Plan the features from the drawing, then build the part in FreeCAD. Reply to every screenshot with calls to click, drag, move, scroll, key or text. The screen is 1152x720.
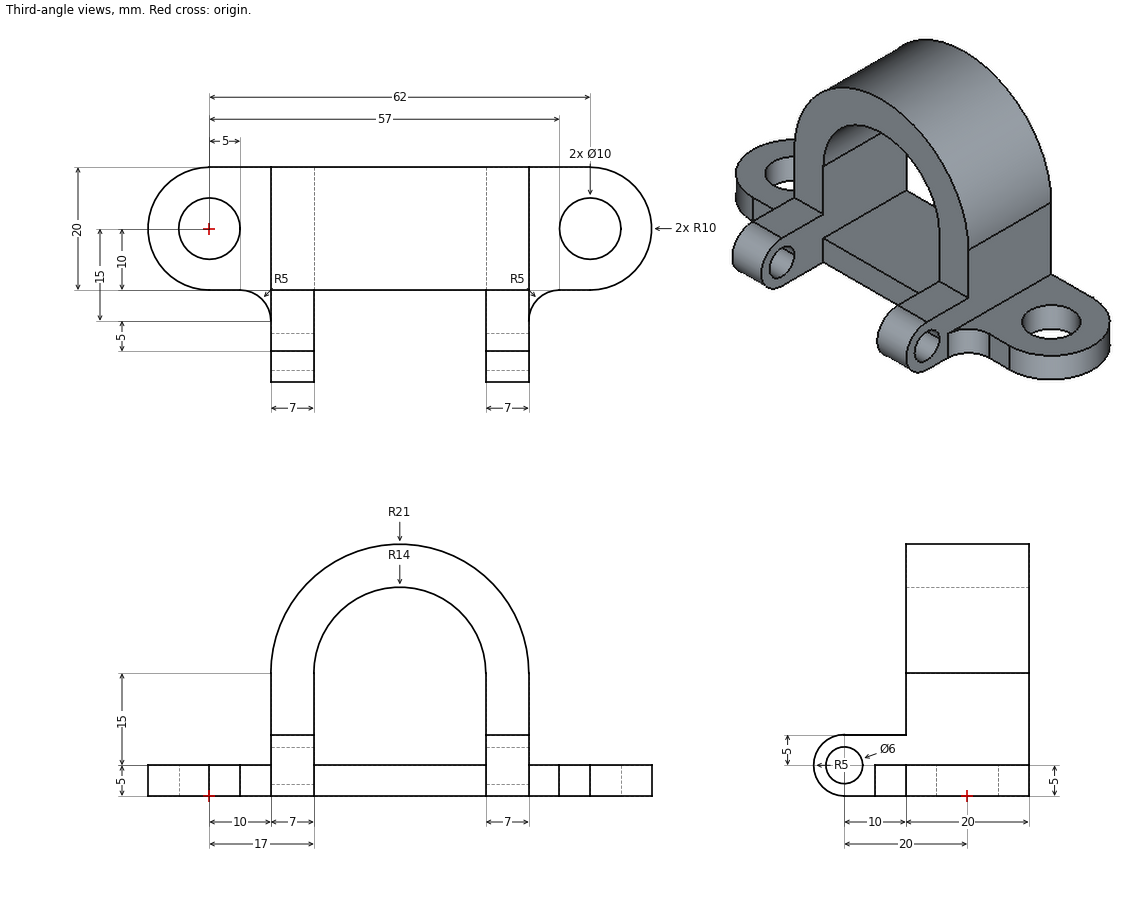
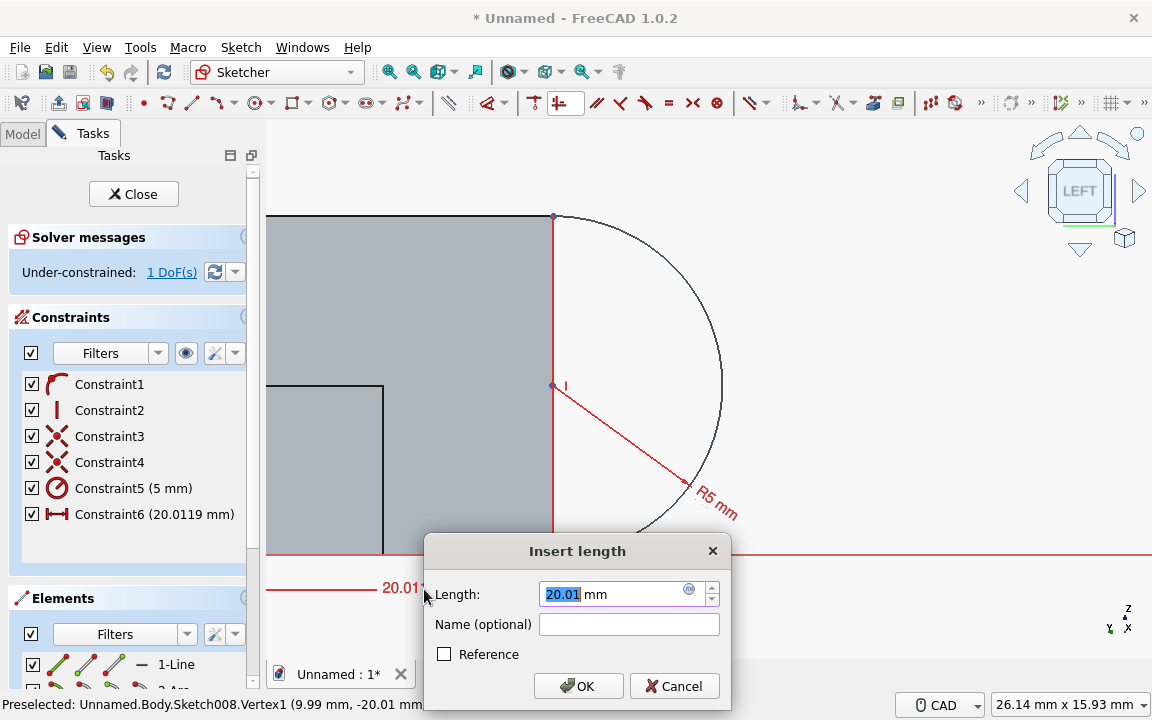
text(20)
key(Return)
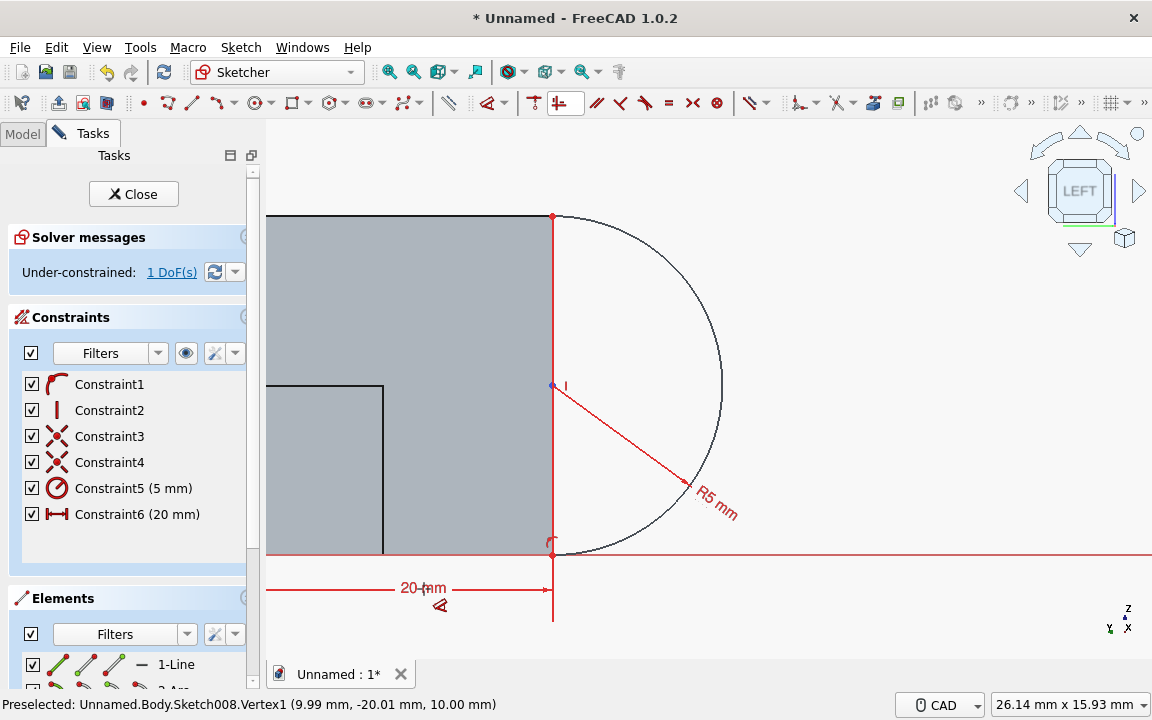
click(553, 386)
click(333, 589)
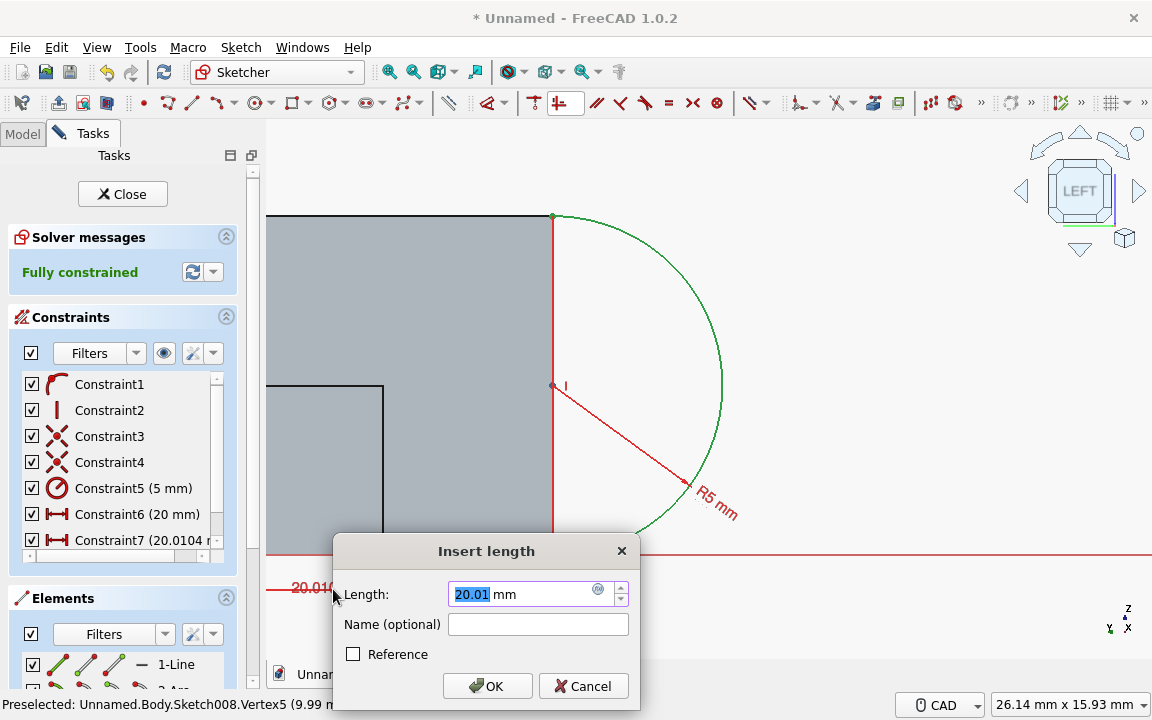
text(20)
key(Return)
key(Escape)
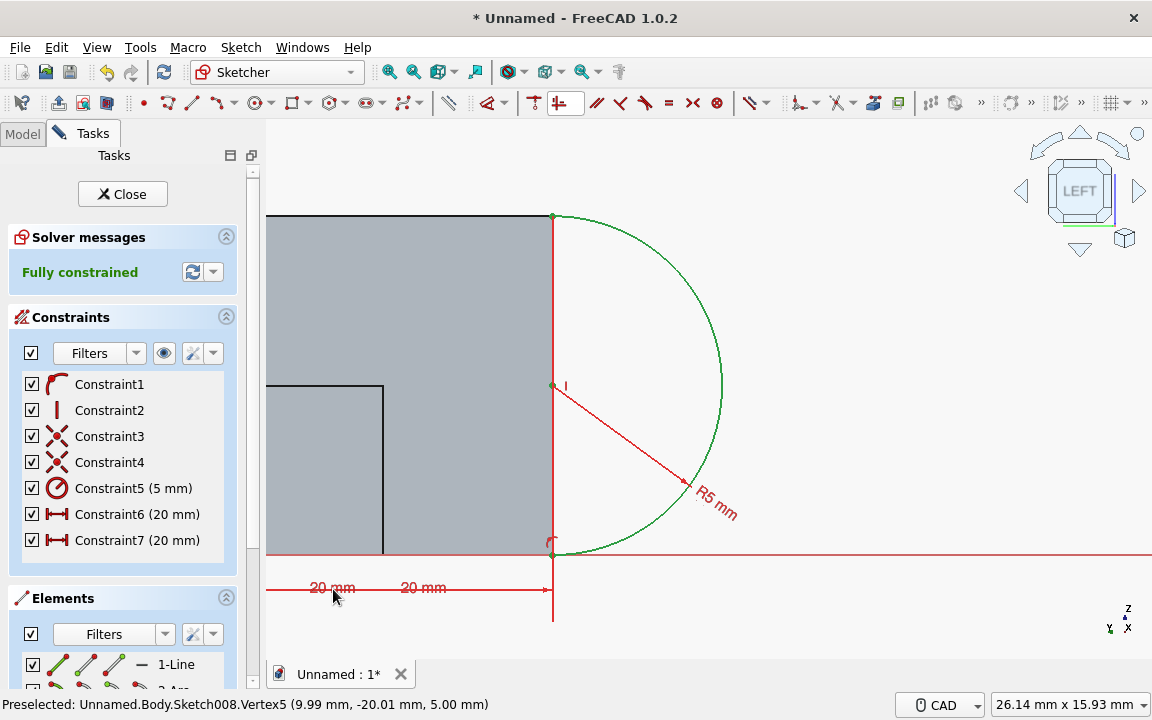
click(123, 194)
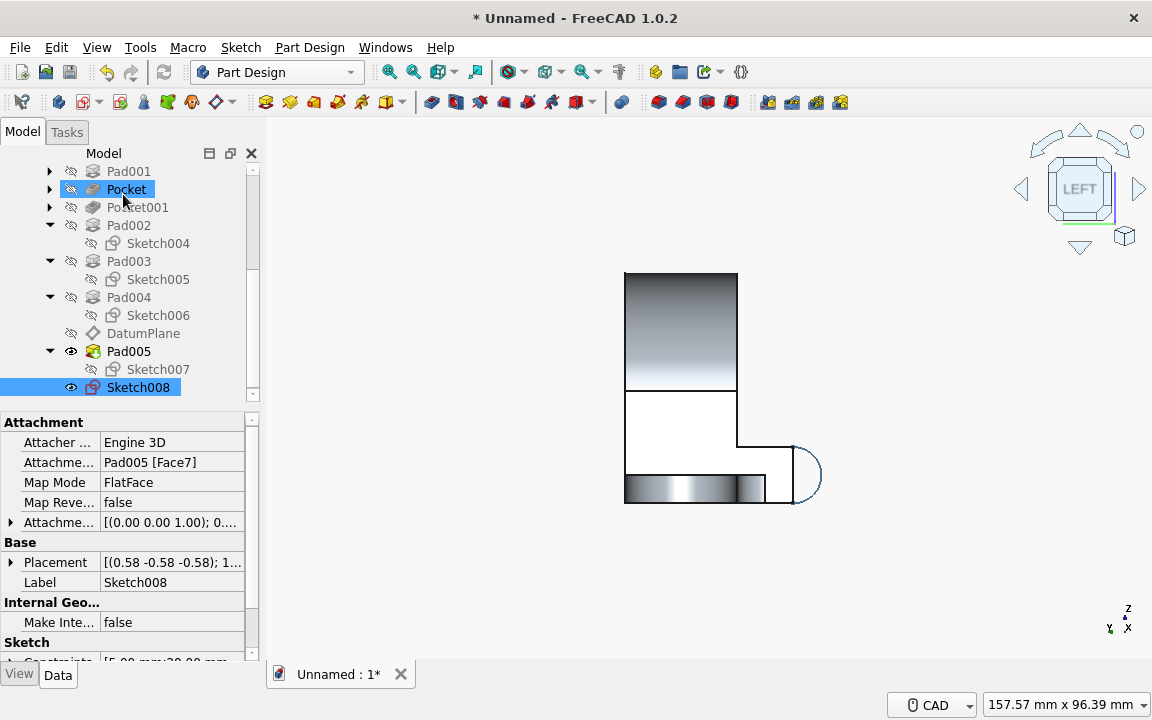
click(266, 102)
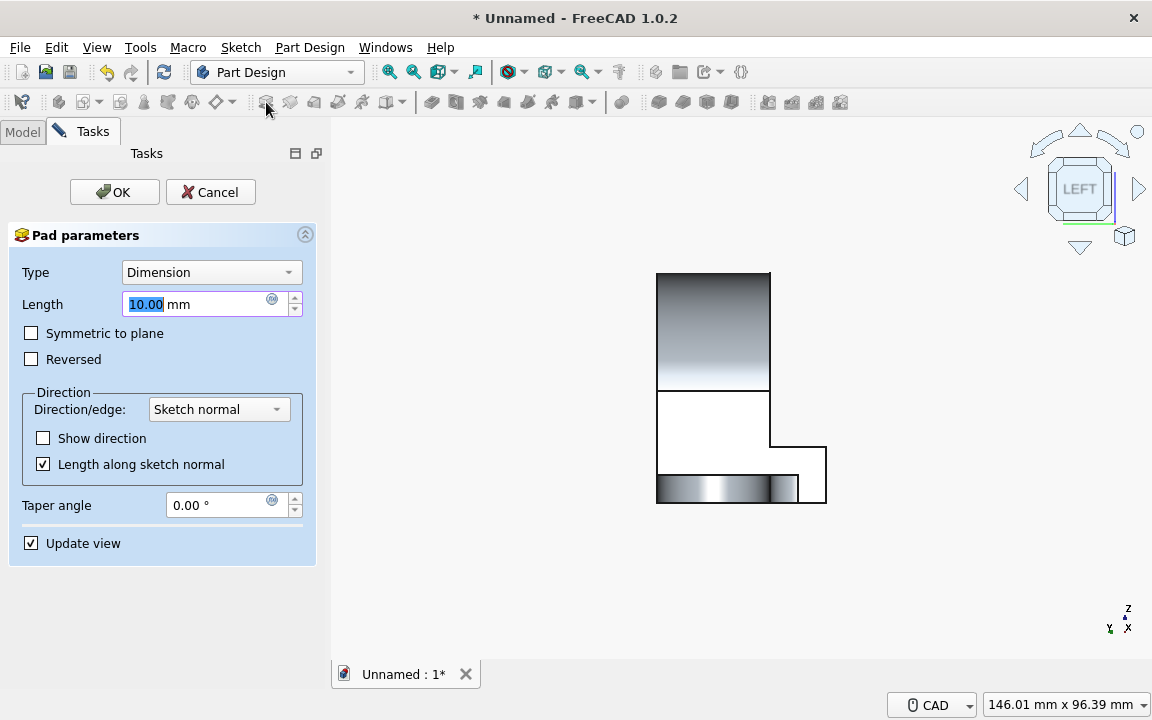
text(7)
key(Tab)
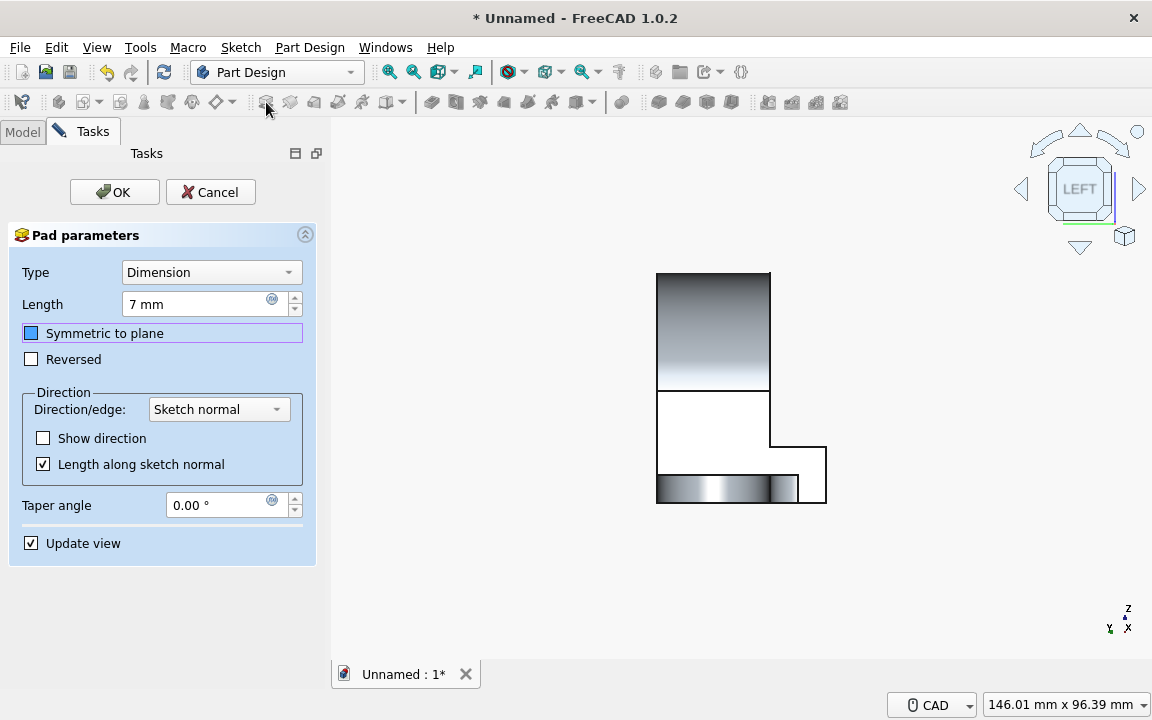
click(30, 359)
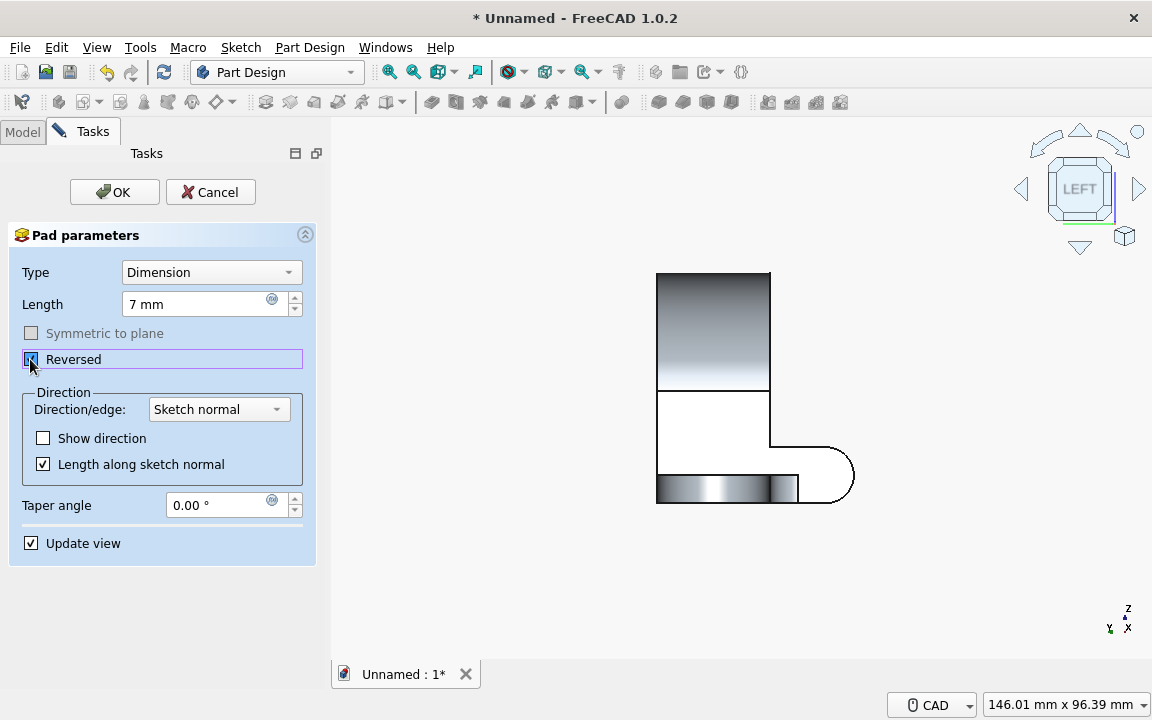
click(115, 192)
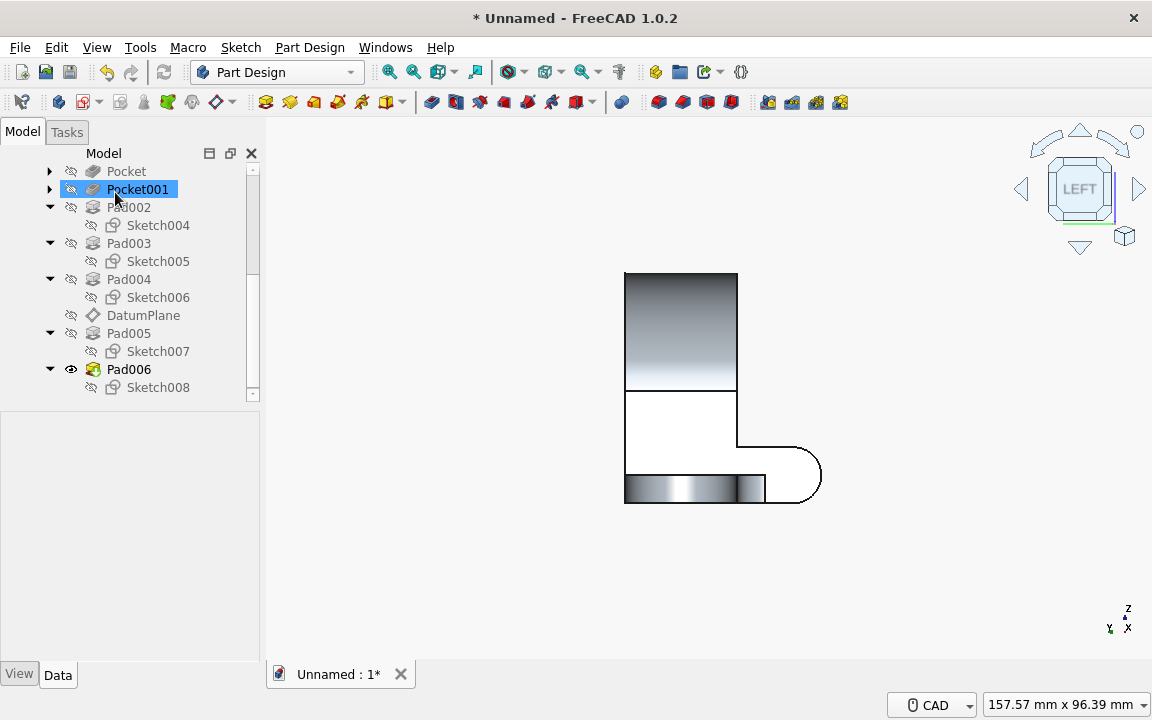
key(v)
key(f)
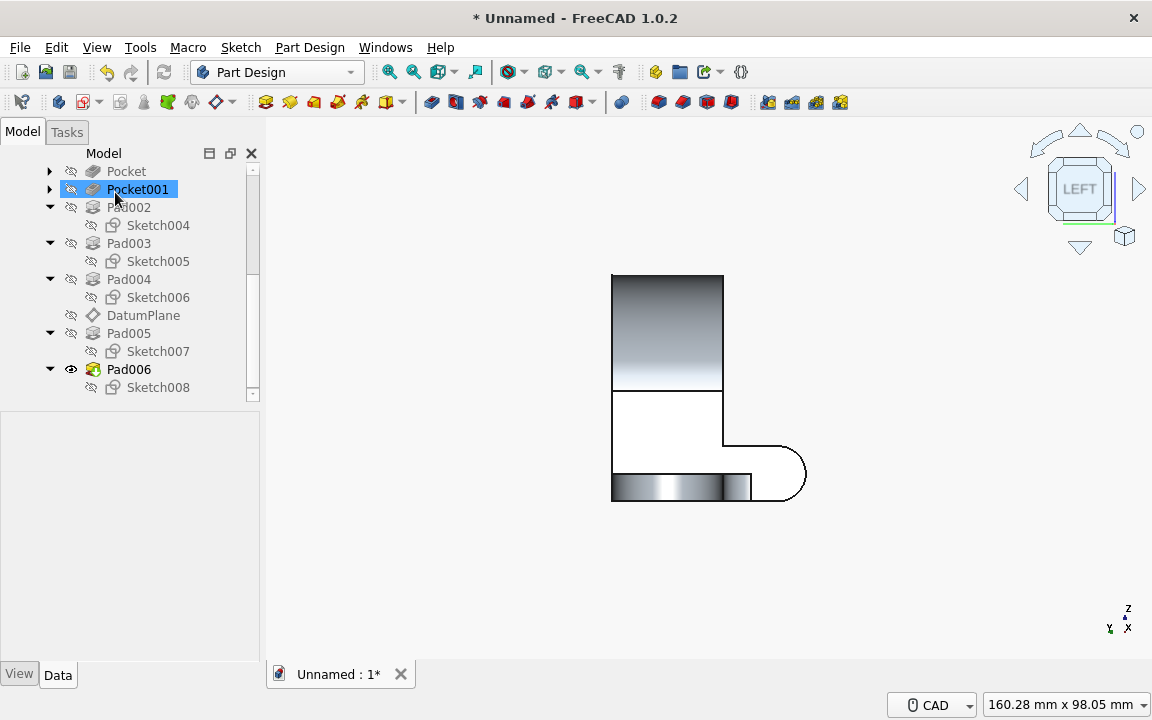
scroll(140, 275, down, 3)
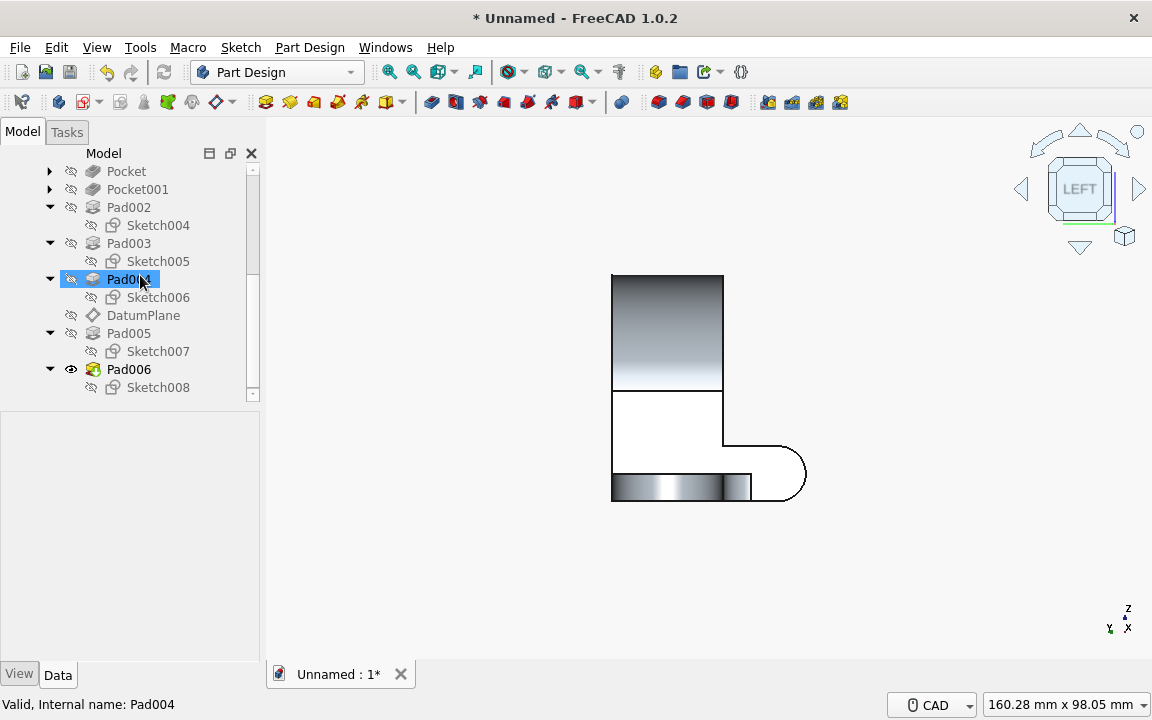
scroll(140, 275, up, 15)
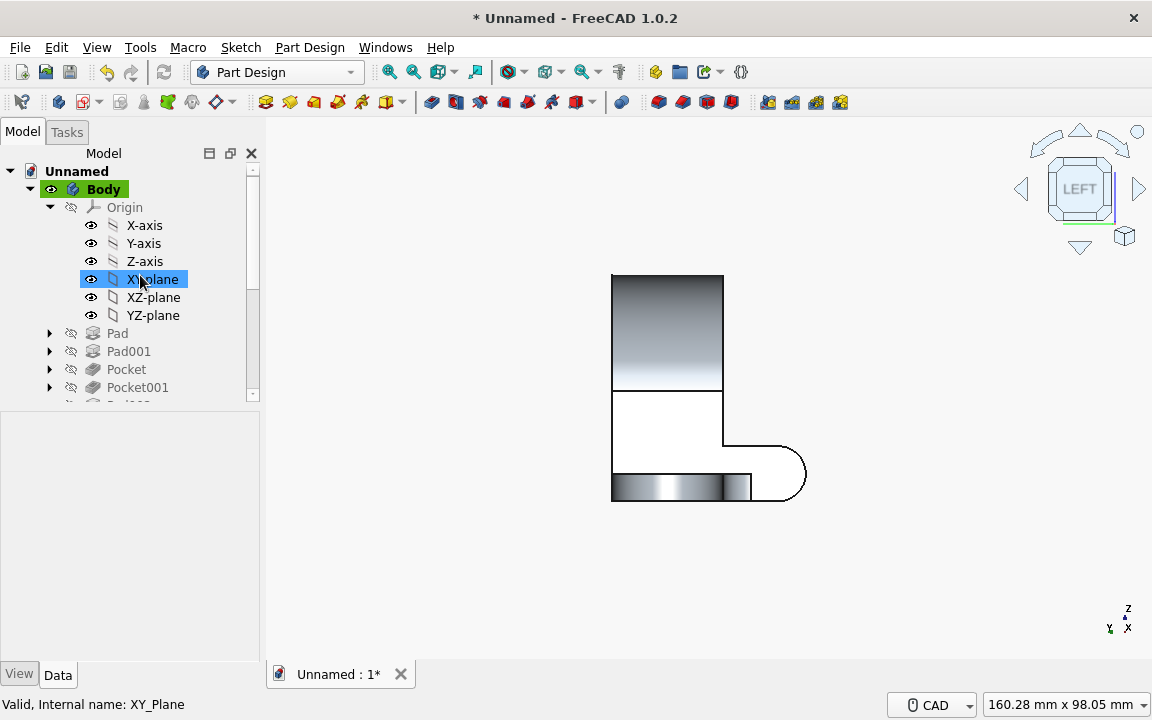
click(136, 315)